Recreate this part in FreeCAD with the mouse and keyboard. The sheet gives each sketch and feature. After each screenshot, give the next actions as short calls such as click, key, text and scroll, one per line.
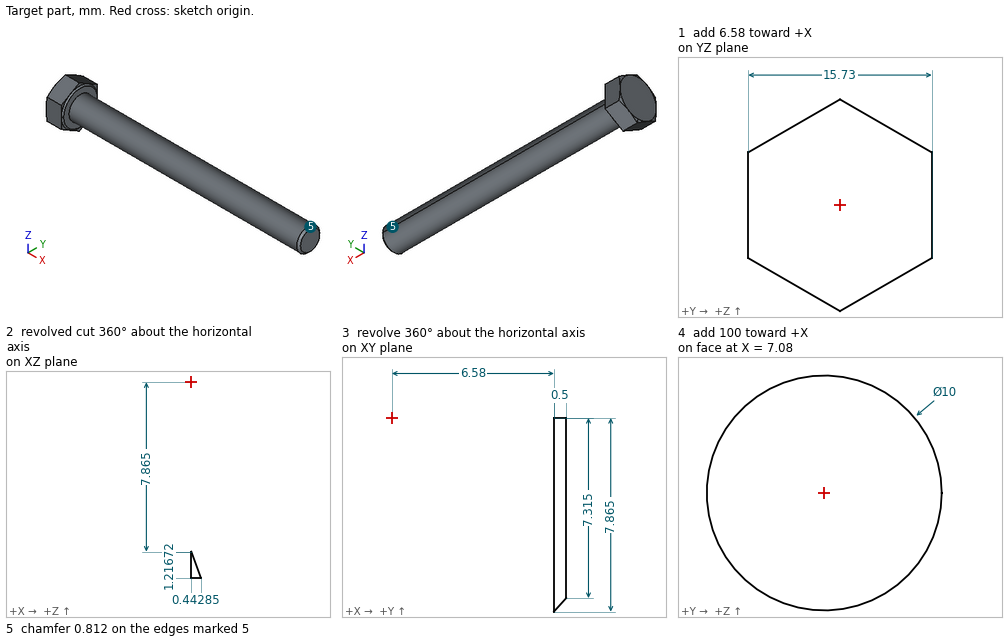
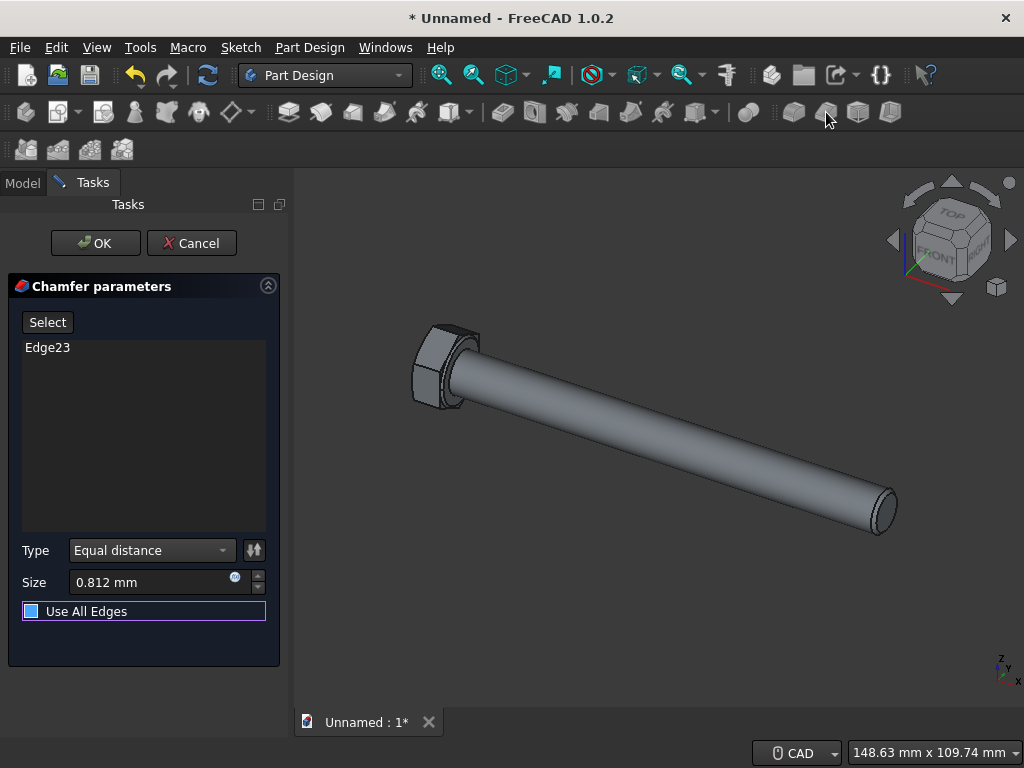
click(96, 243)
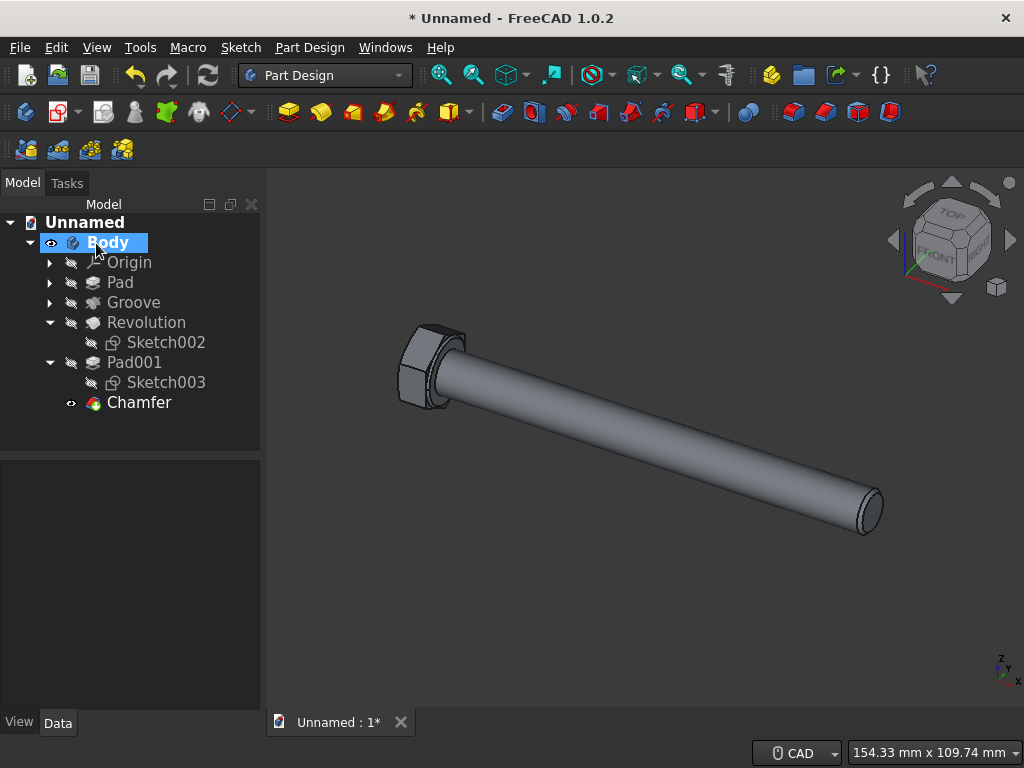
key(0)